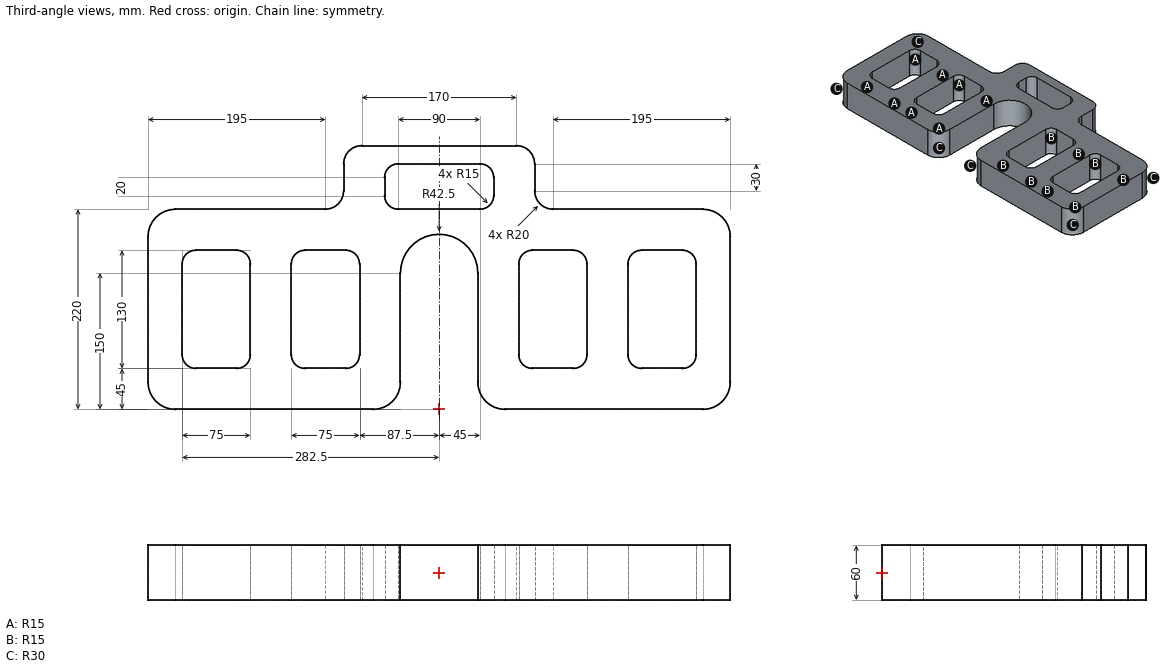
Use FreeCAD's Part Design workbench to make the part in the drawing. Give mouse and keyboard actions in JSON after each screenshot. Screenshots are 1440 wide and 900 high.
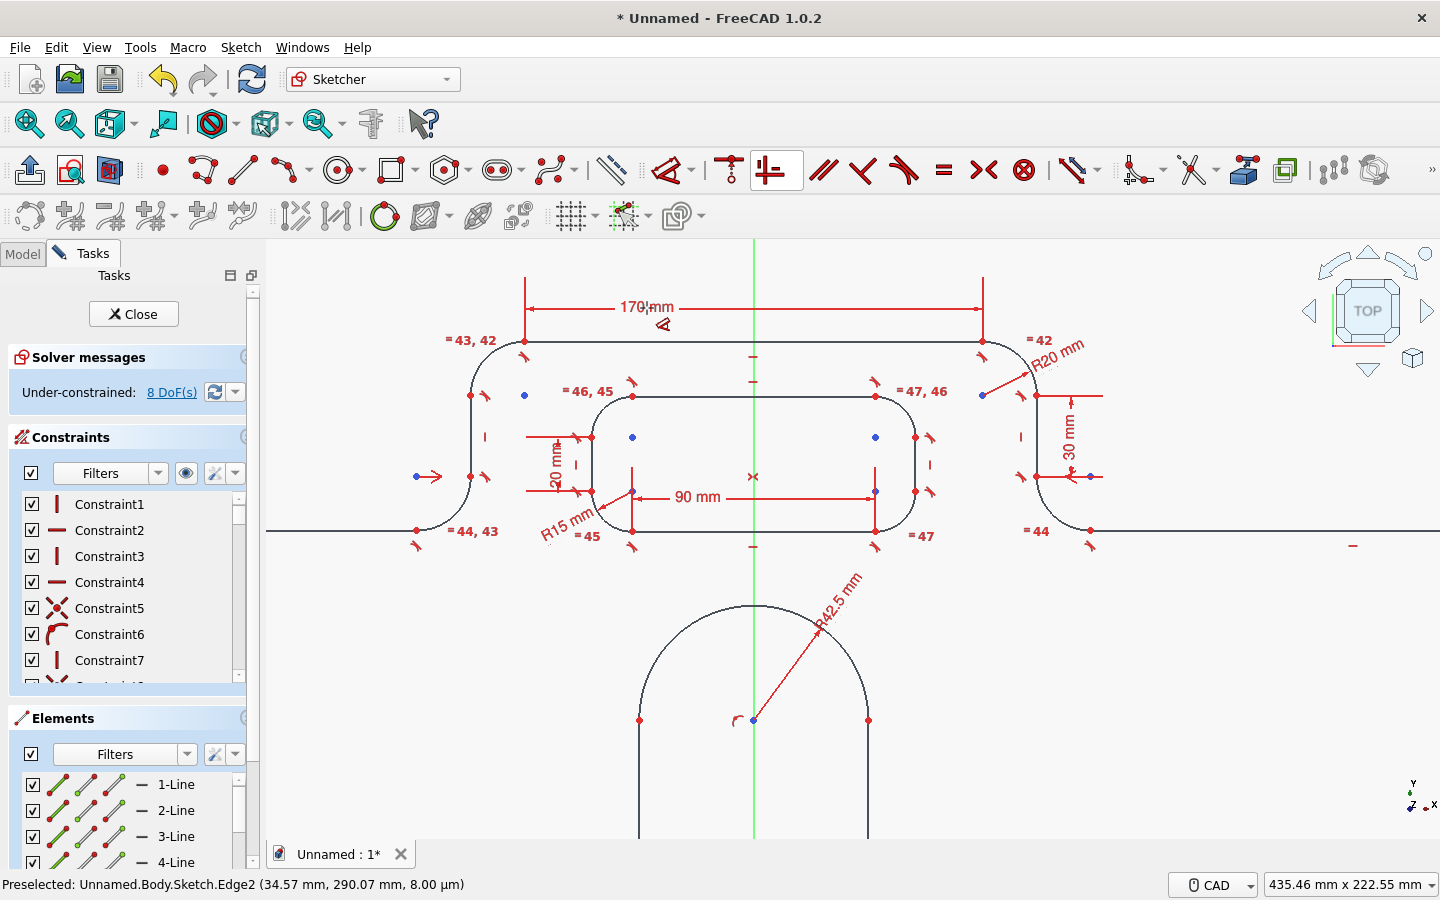
{"action": "left_click", "coordinate": [312, 531]}
{"action": "left_click", "coordinate": [355, 497]}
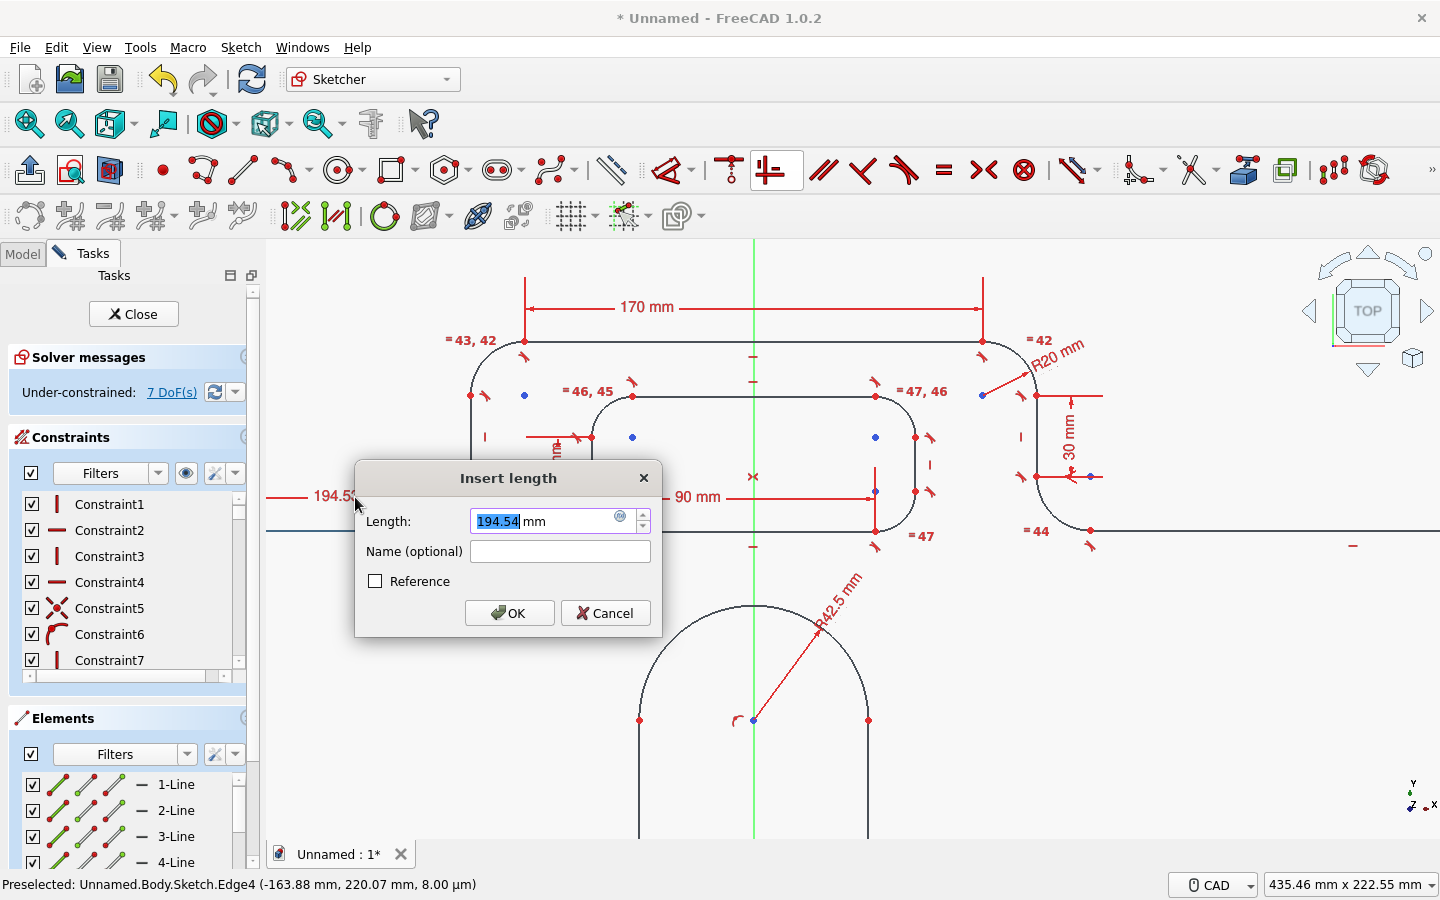
{"action": "type", "text": "195"}
{"action": "key", "text": "Return"}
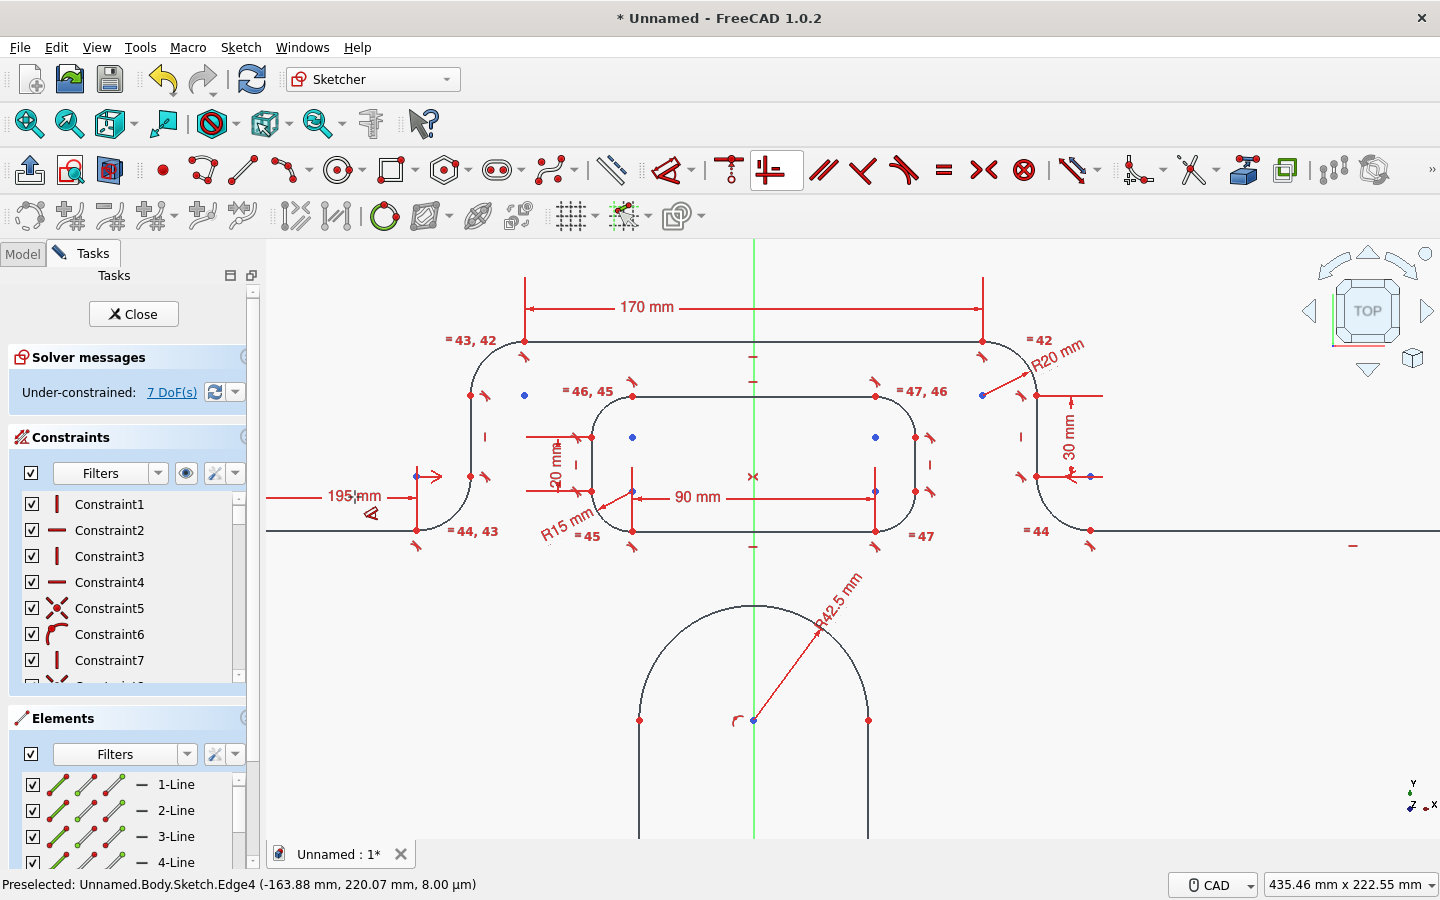
{"action": "scroll", "coordinate": [802, 426], "scroll_direction": "down", "scroll_amount": 5}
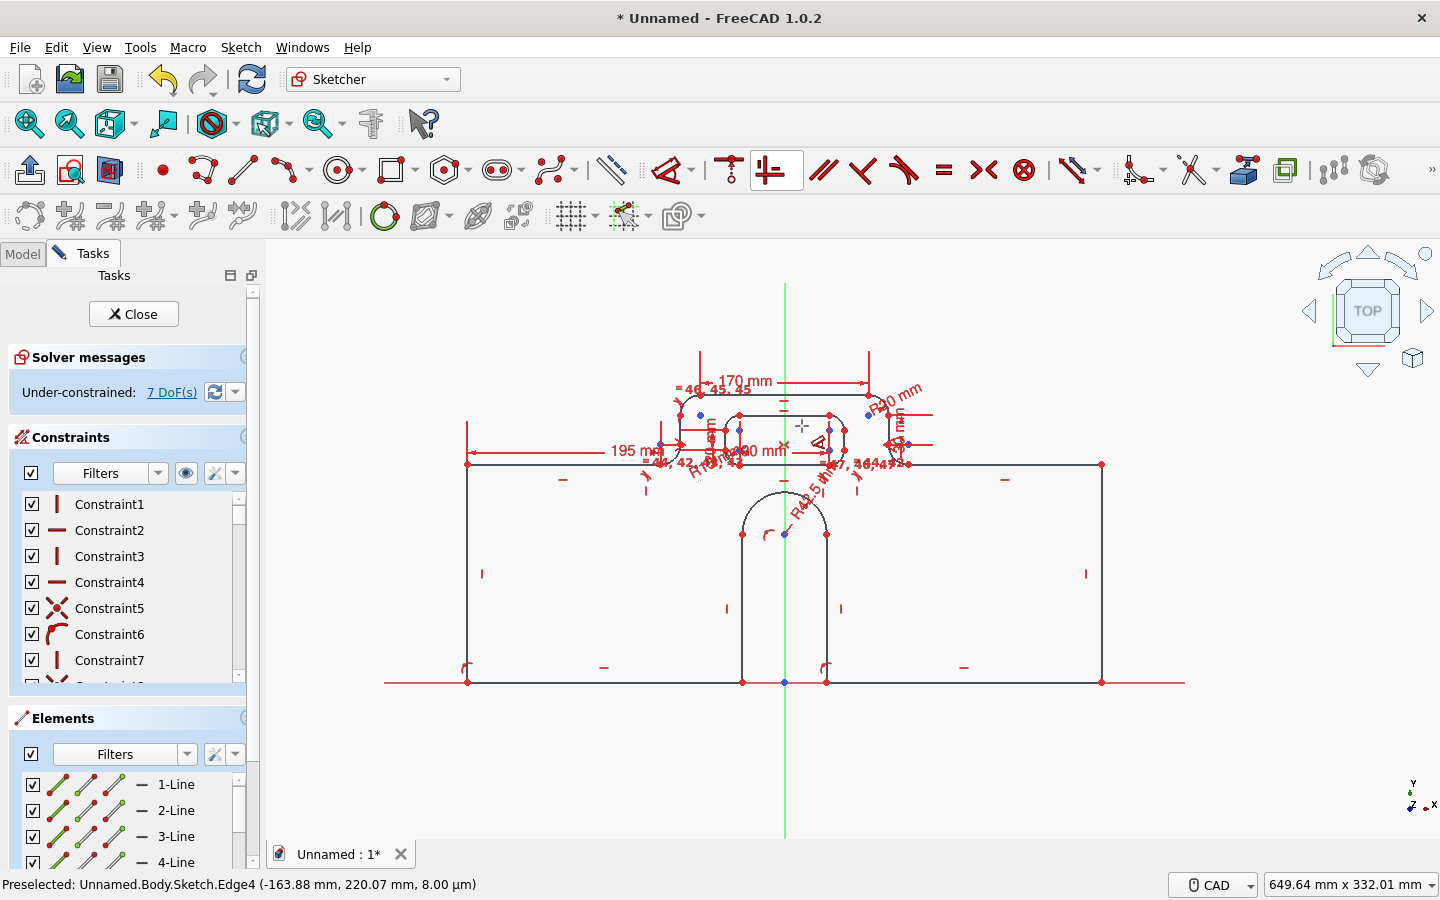
{"action": "left_click", "coordinate": [467, 530]}
{"action": "left_click", "coordinate": [433, 574]}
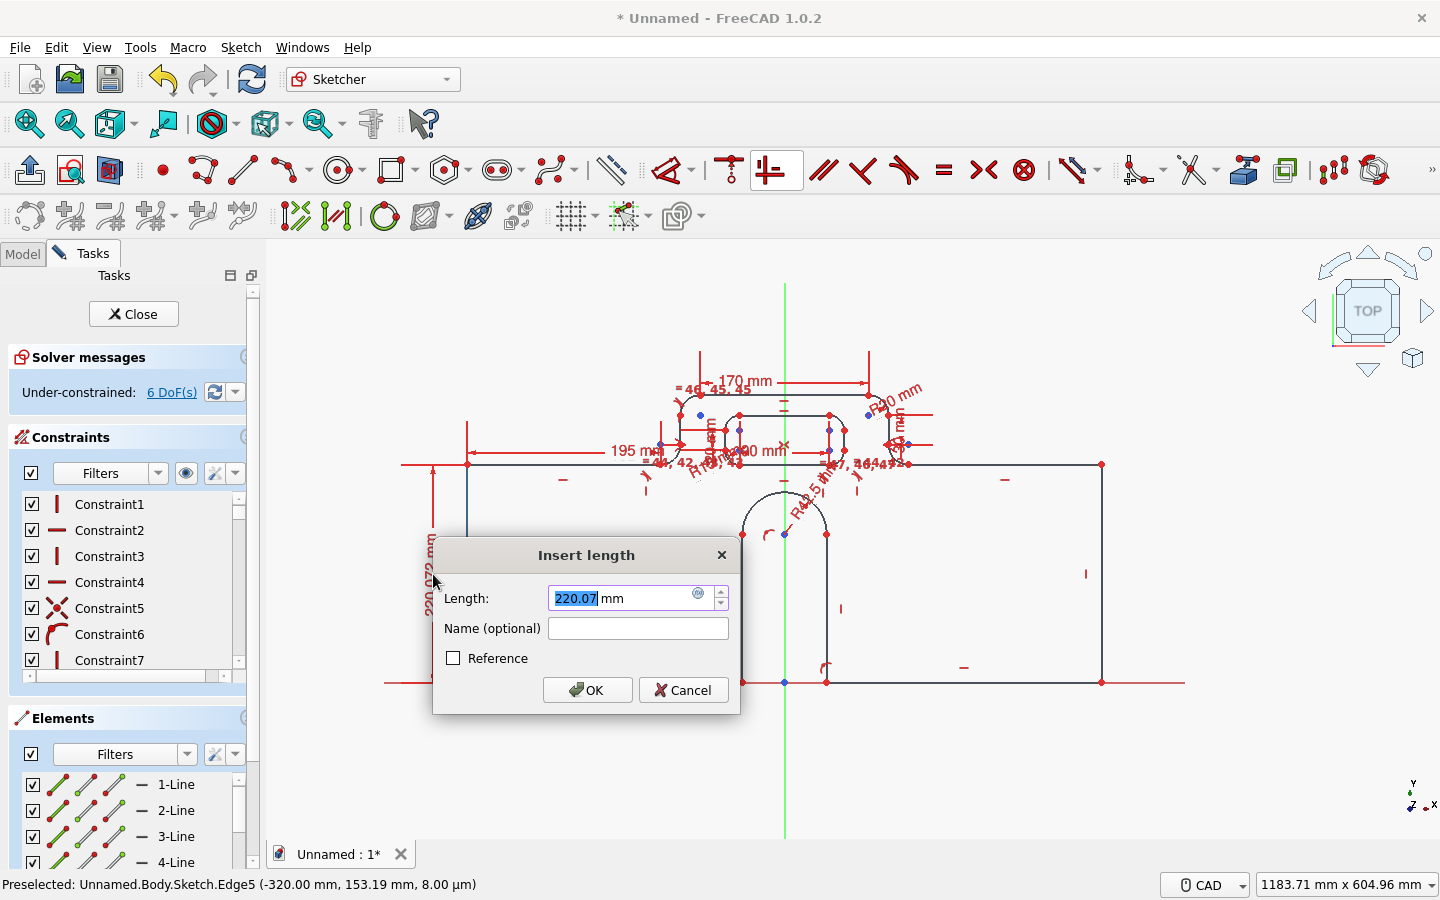
{"action": "type", "text": "220"}
{"action": "key", "text": "Return"}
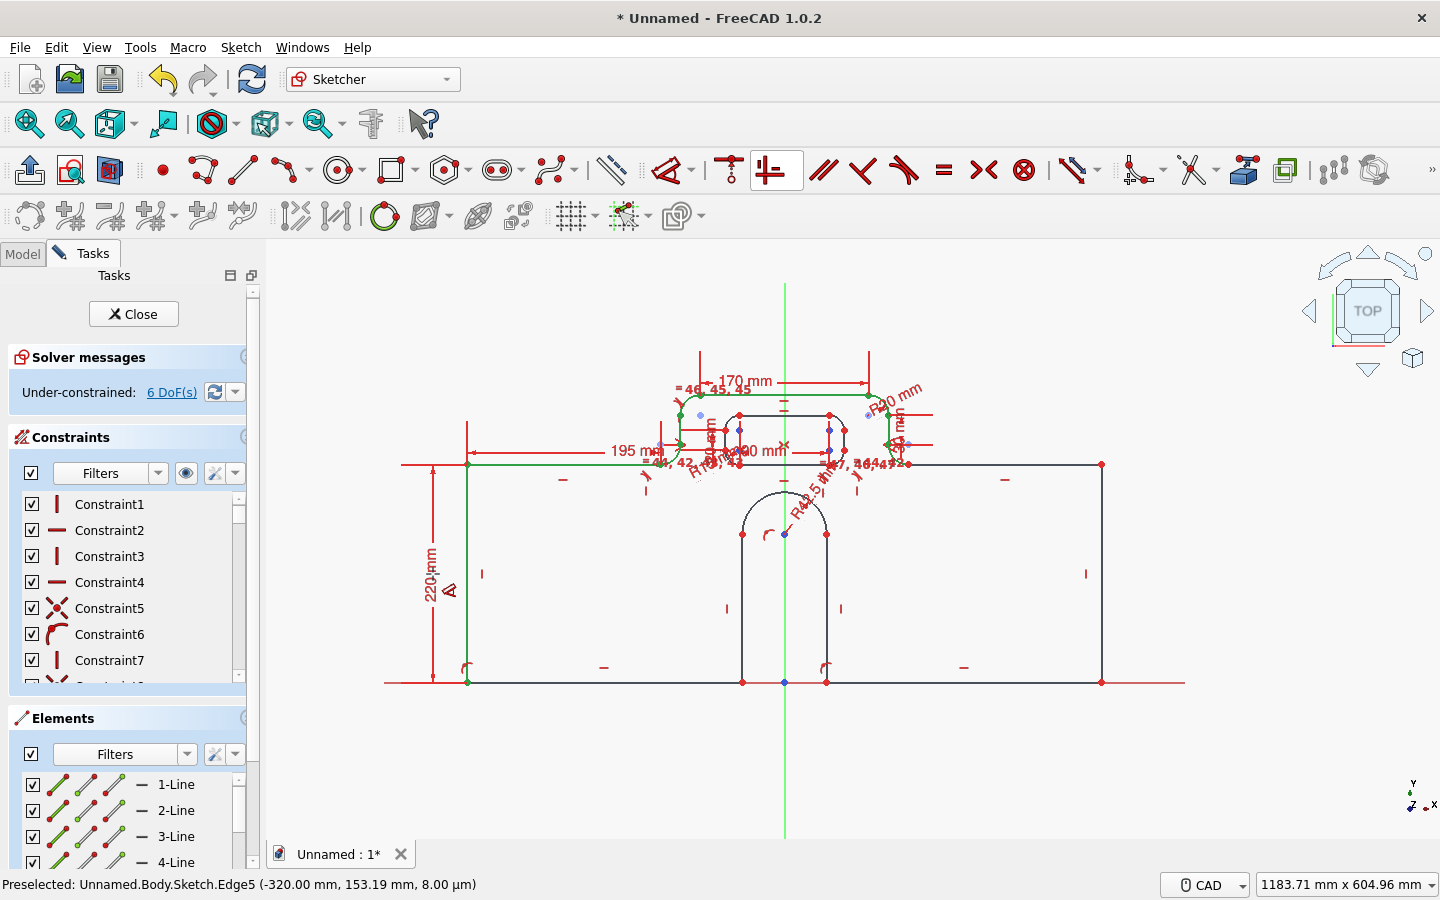
{"action": "left_click", "coordinate": [742, 638]}
{"action": "left_click", "coordinate": [708, 609]}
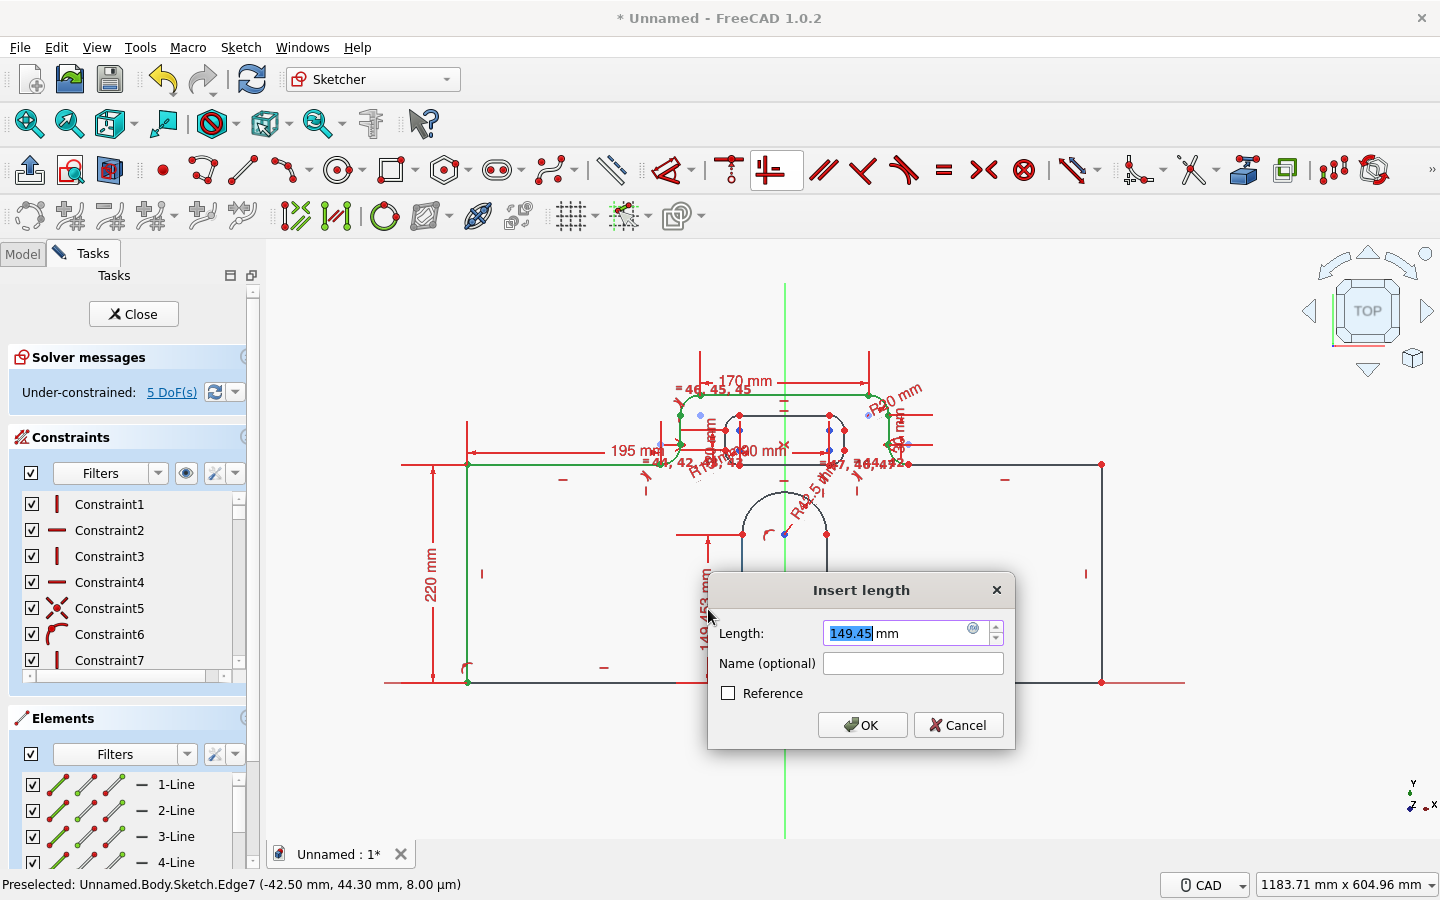
{"action": "type", "text": "150"}
{"action": "key", "text": "Return"}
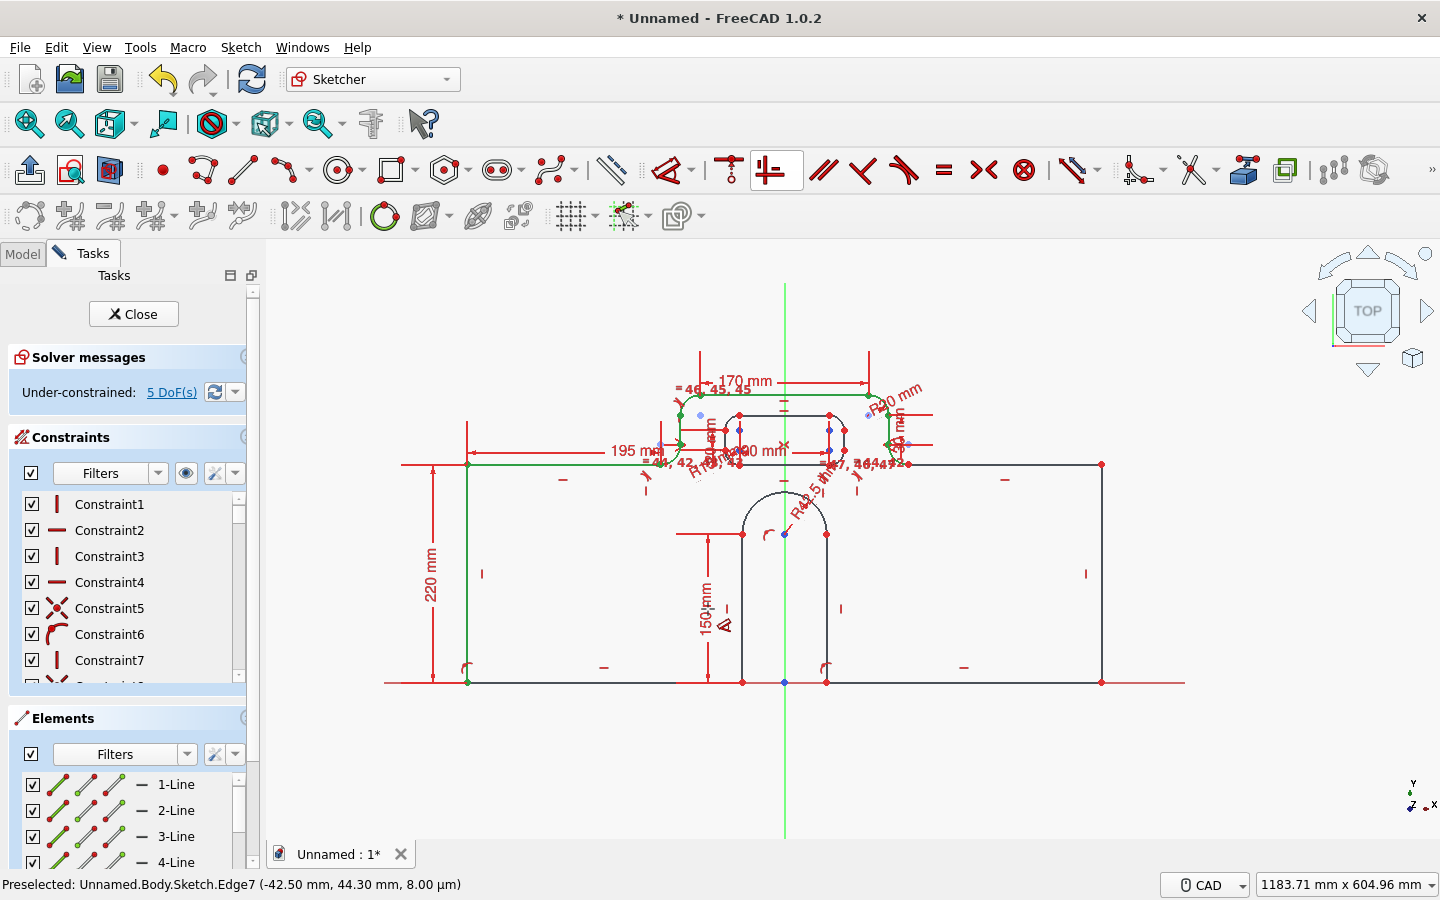
{"action": "left_click", "coordinate": [827, 579]}
{"action": "left_click", "coordinate": [861, 609]}